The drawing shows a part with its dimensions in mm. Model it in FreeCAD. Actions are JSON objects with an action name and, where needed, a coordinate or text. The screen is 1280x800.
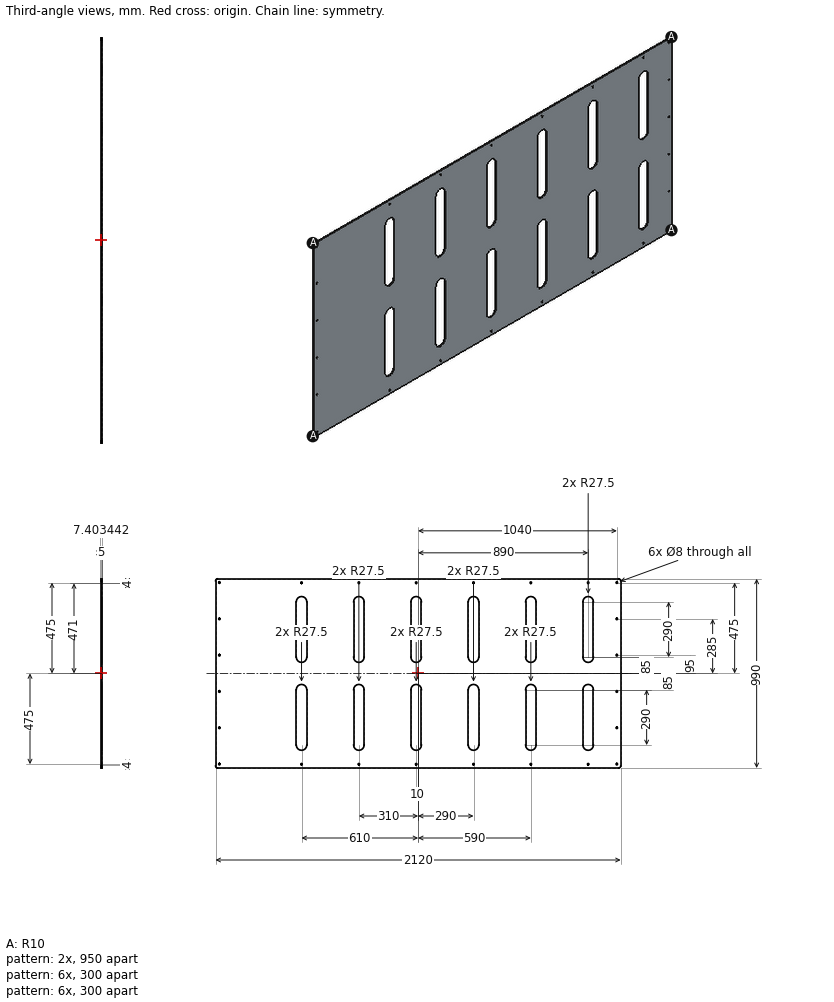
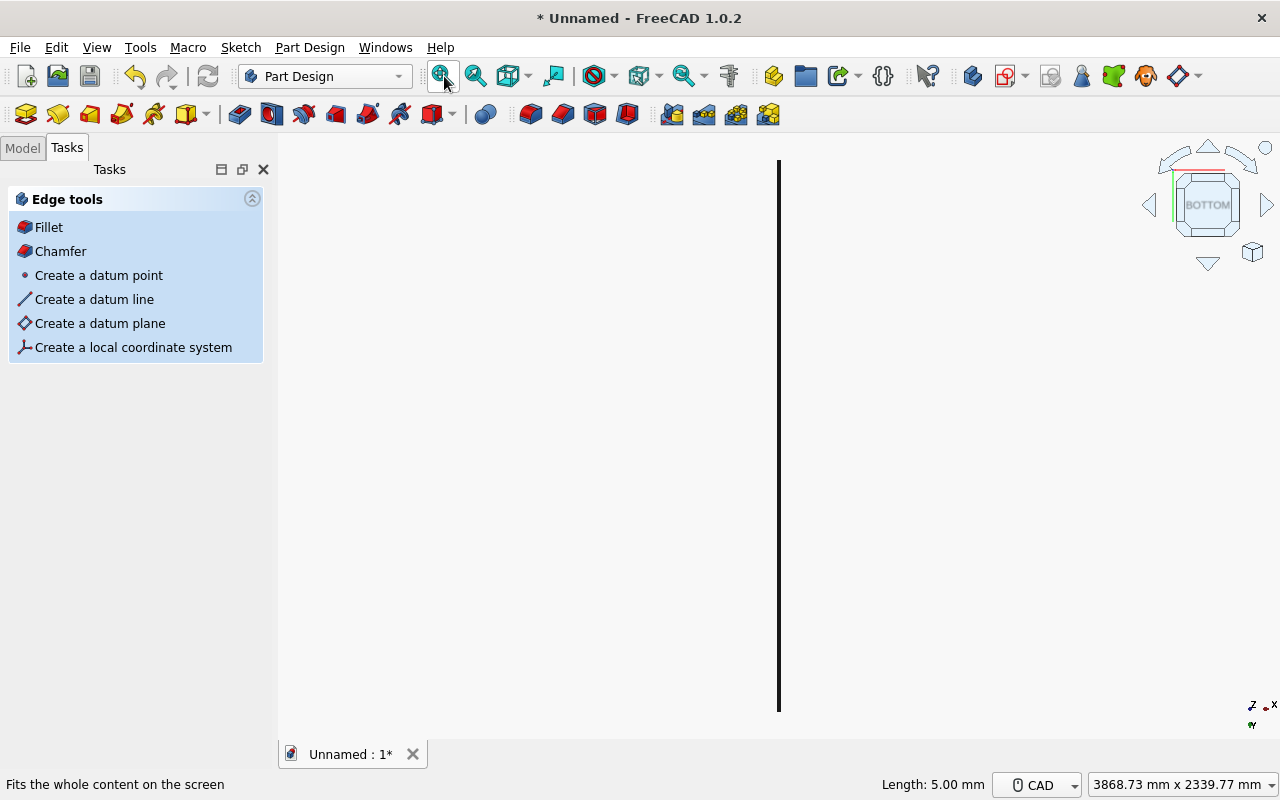
{"action": "key", "text": "4"}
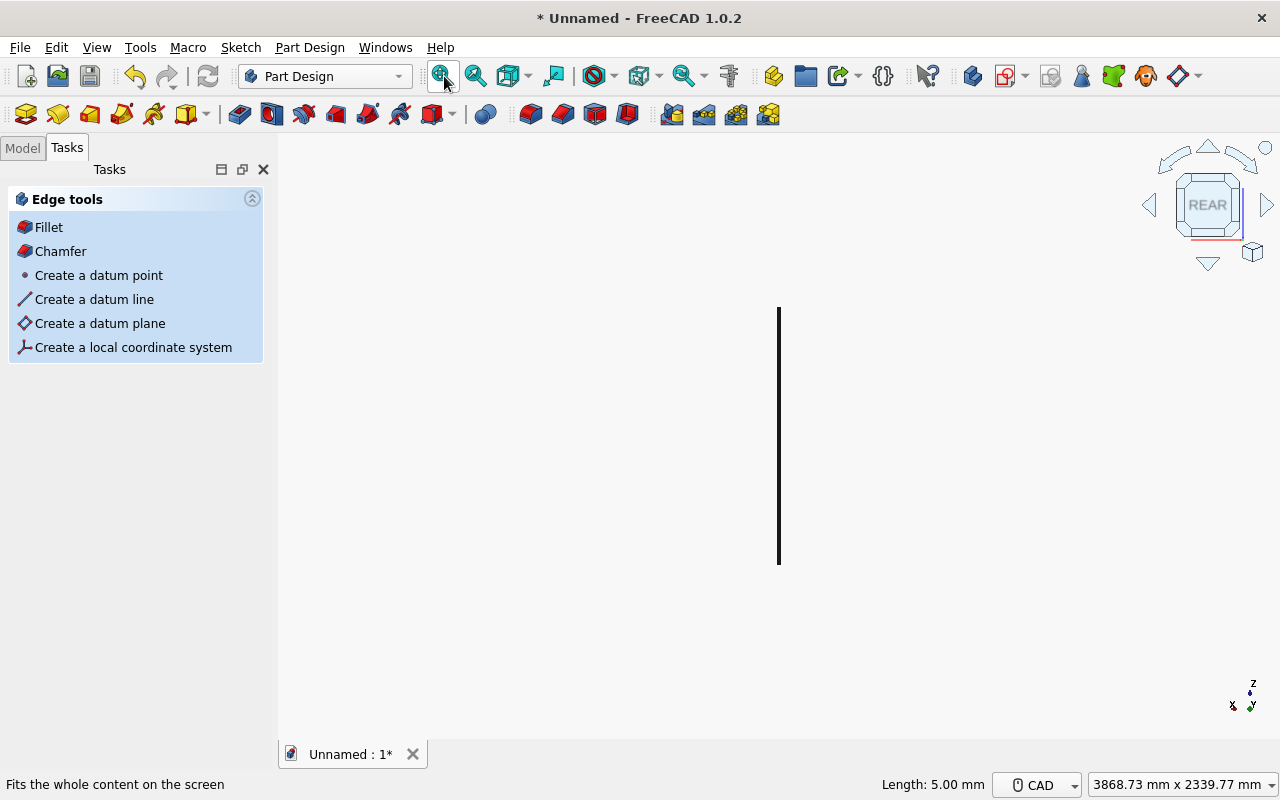
{"action": "left_click", "coordinate": [444, 76]}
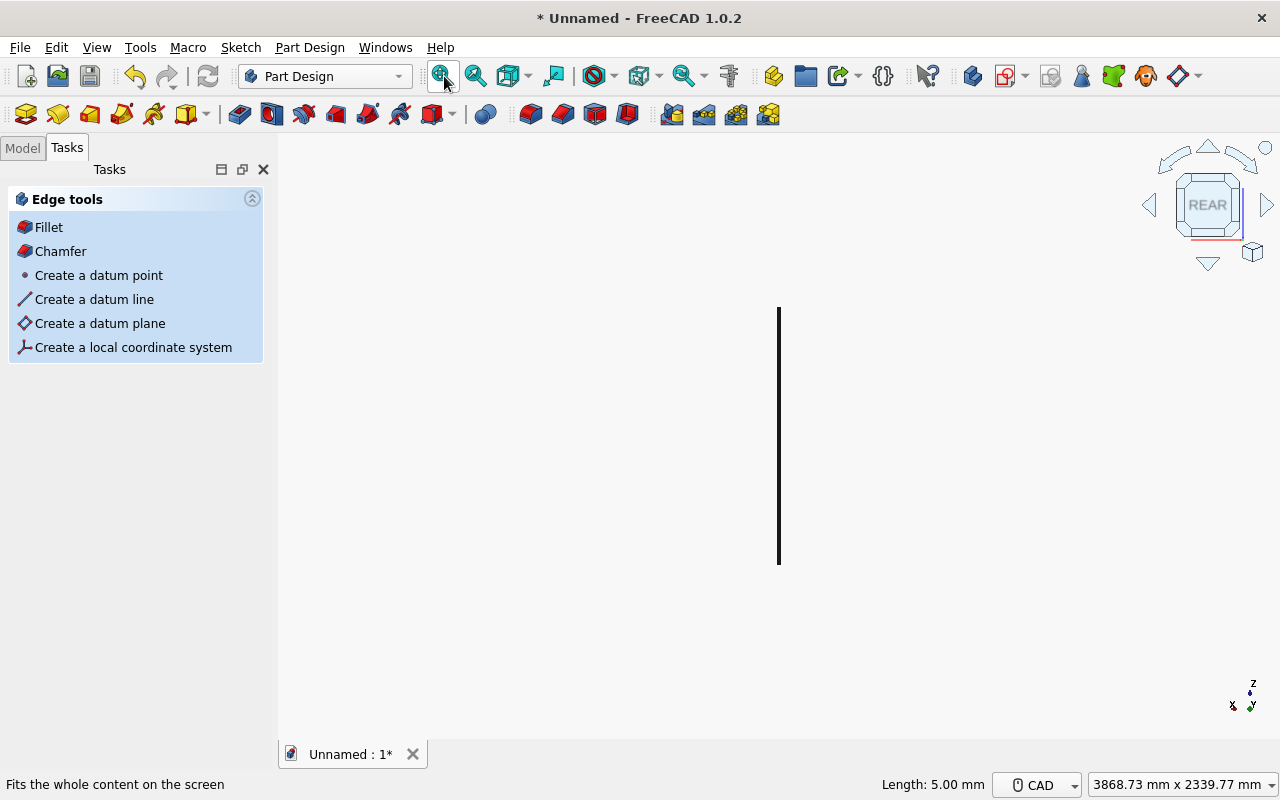
{"action": "scroll", "coordinate": [779, 307], "scroll_direction": "up", "scroll_amount": 15}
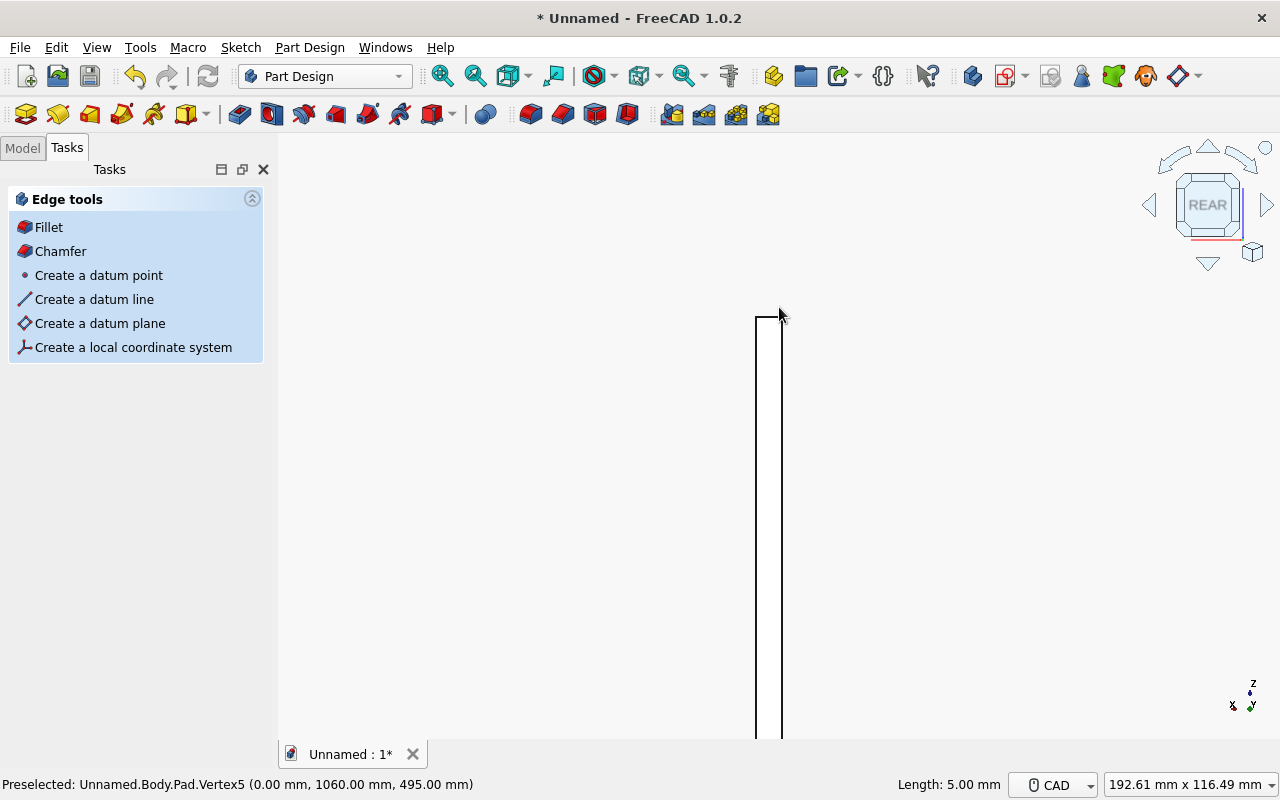
{"action": "left_click", "coordinate": [769, 316], "text": "ctrl"}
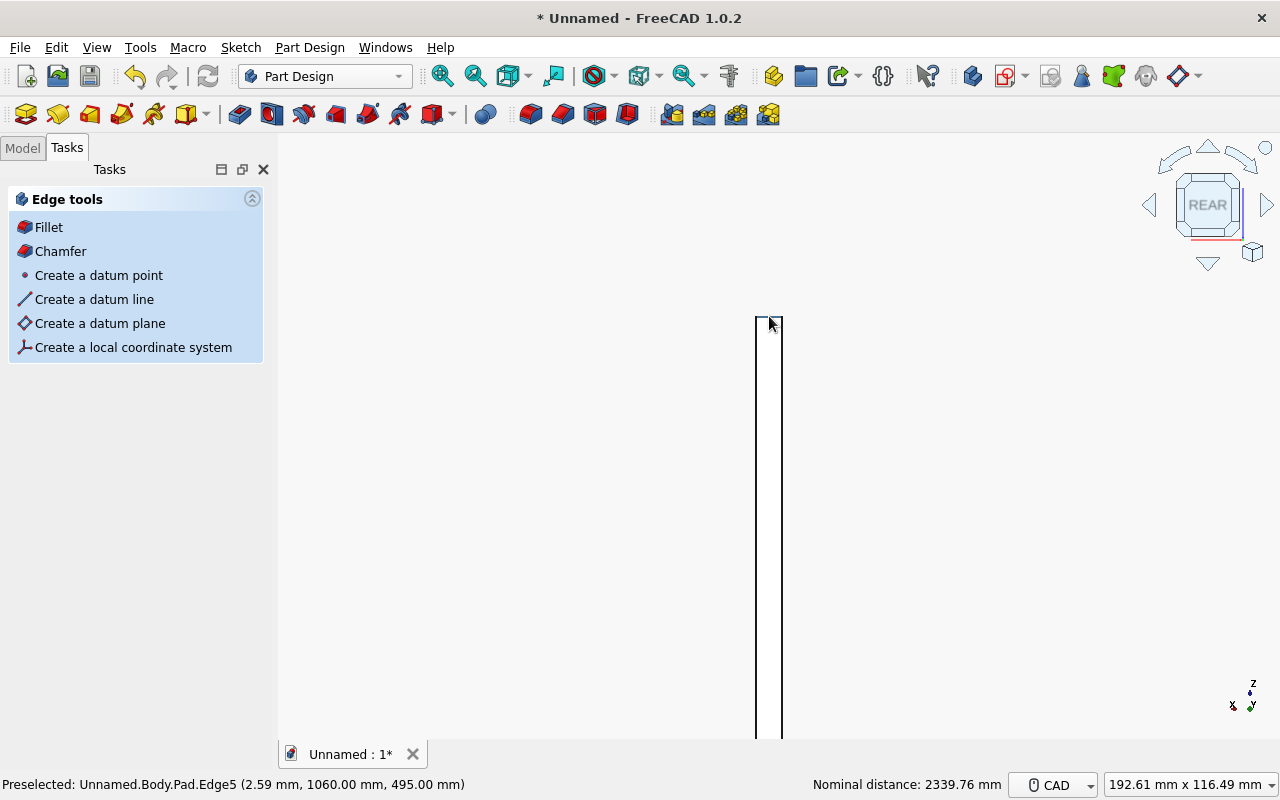
{"action": "left_click", "coordinate": [444, 76]}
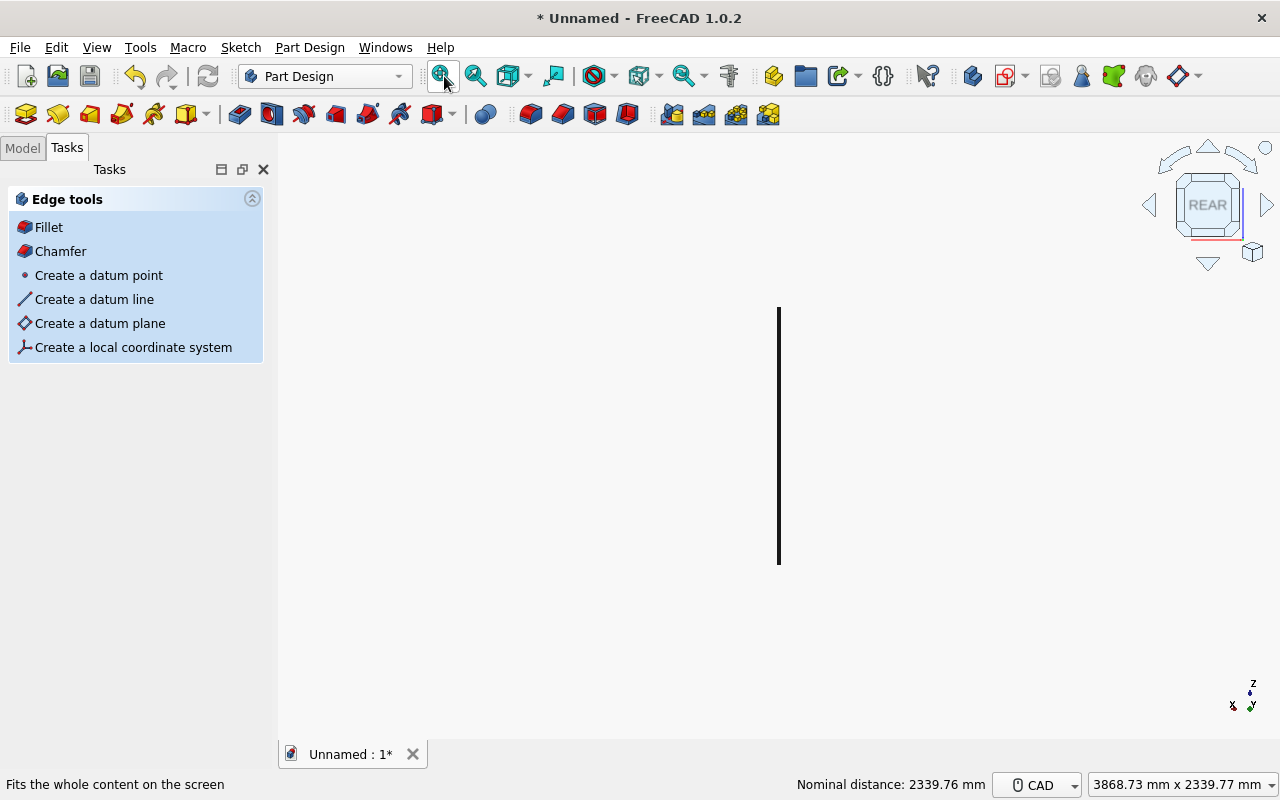
{"action": "key", "text": "6"}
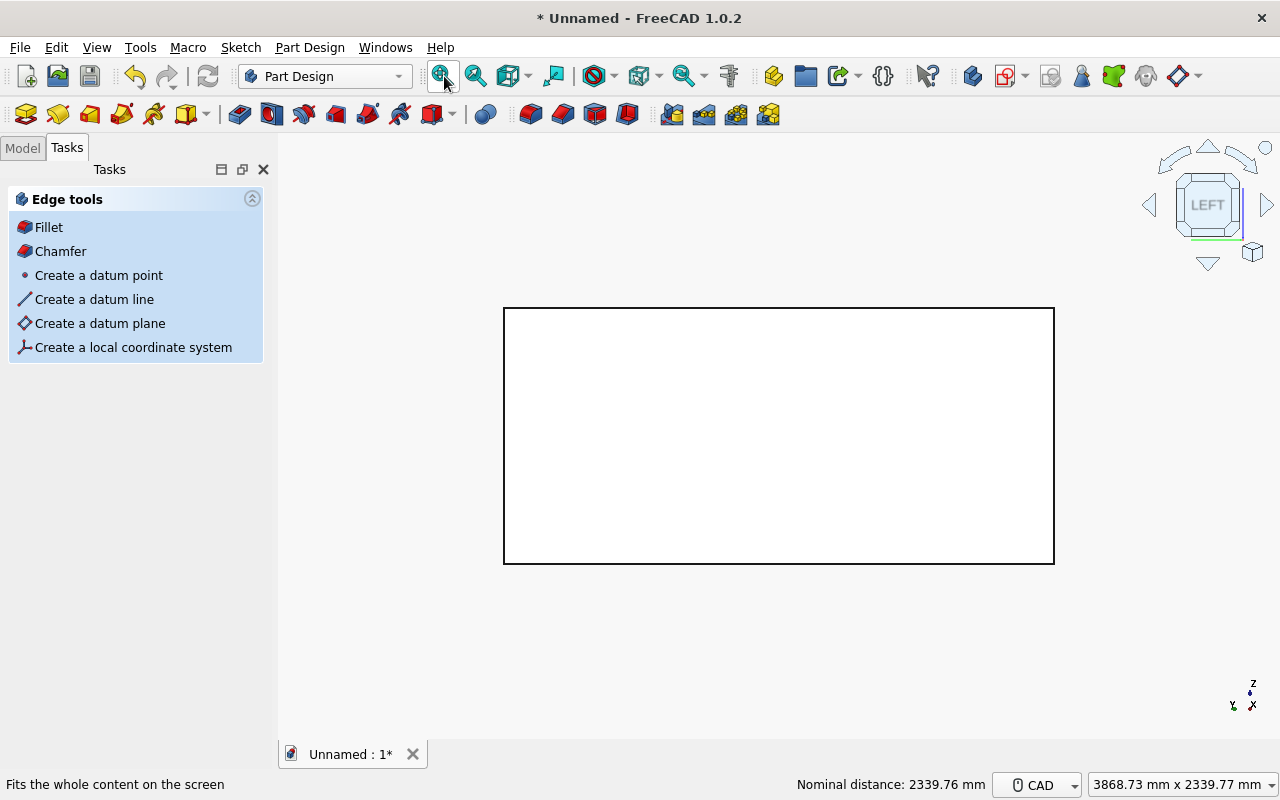
{"action": "scroll", "coordinate": [1054, 307], "scroll_direction": "up", "scroll_amount": 15}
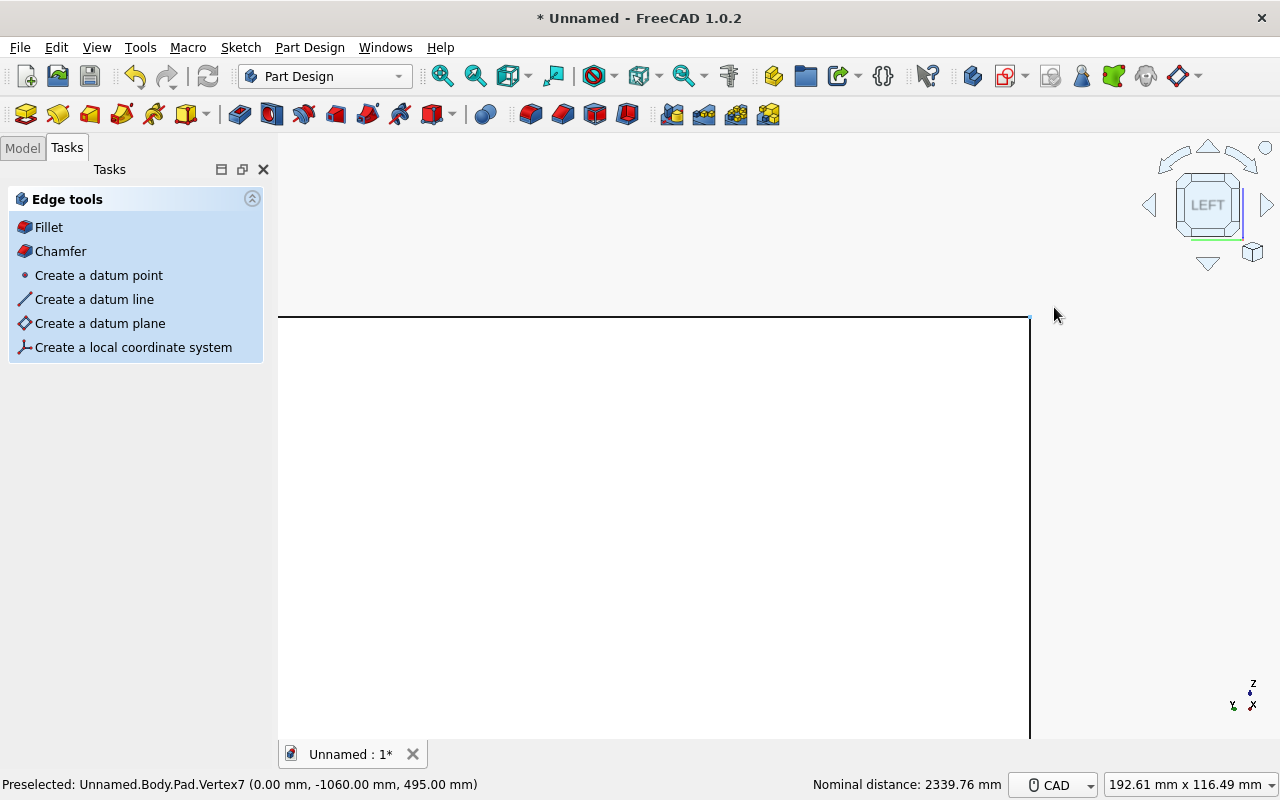
{"action": "left_click", "coordinate": [444, 76]}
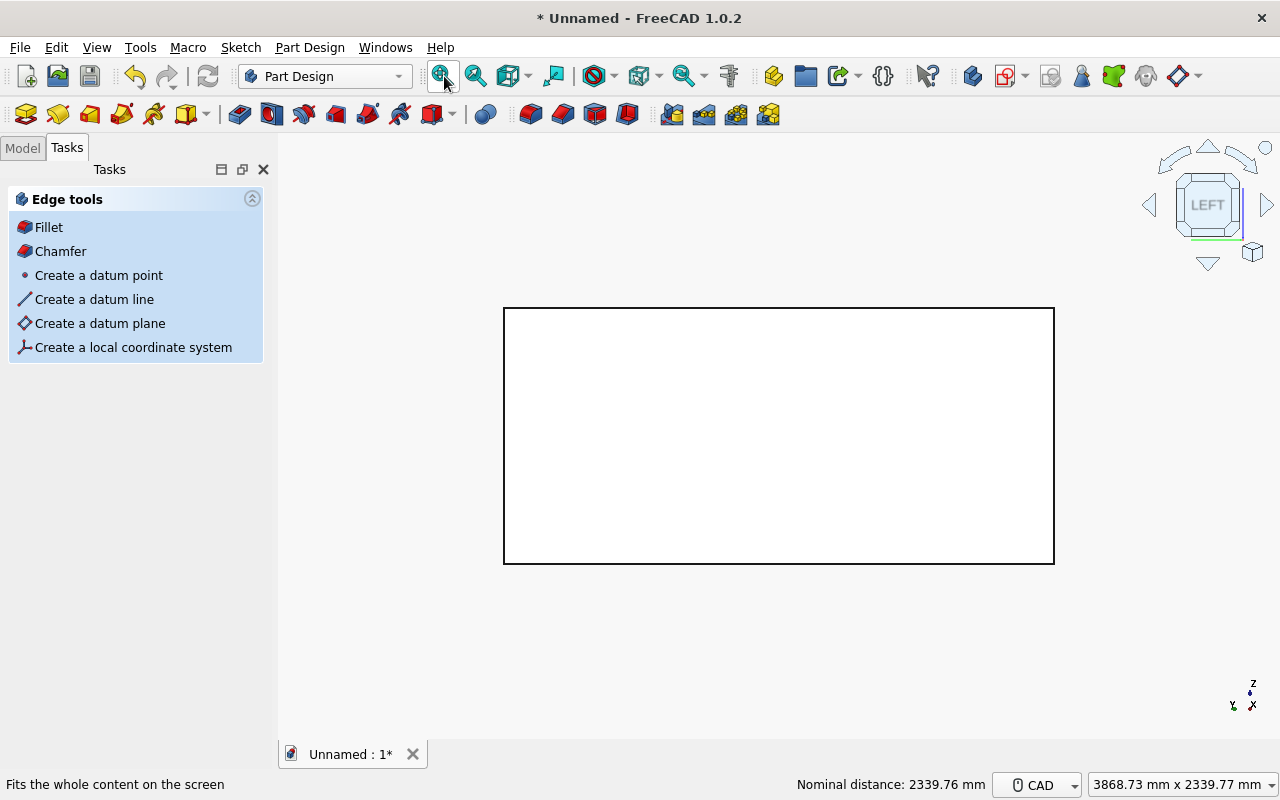
{"action": "key", "text": "v 3"}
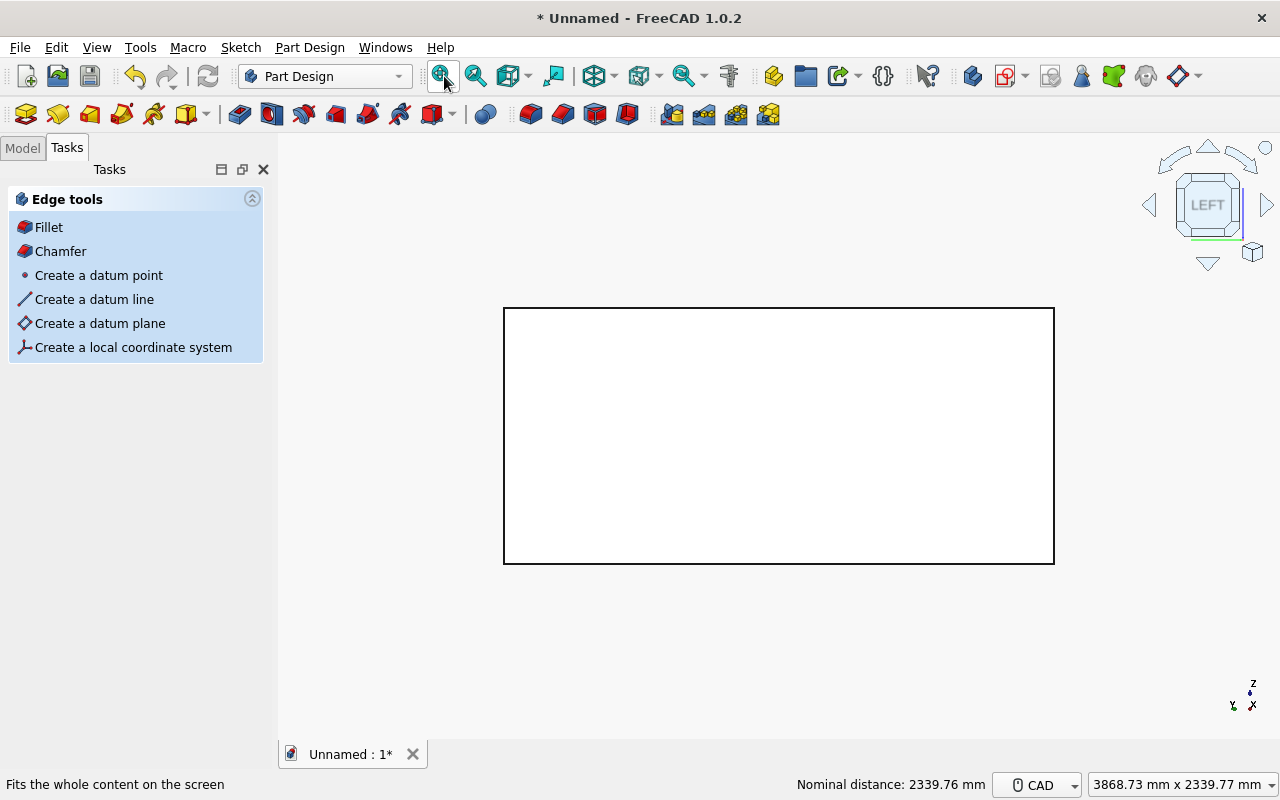
{"action": "key", "text": "0"}